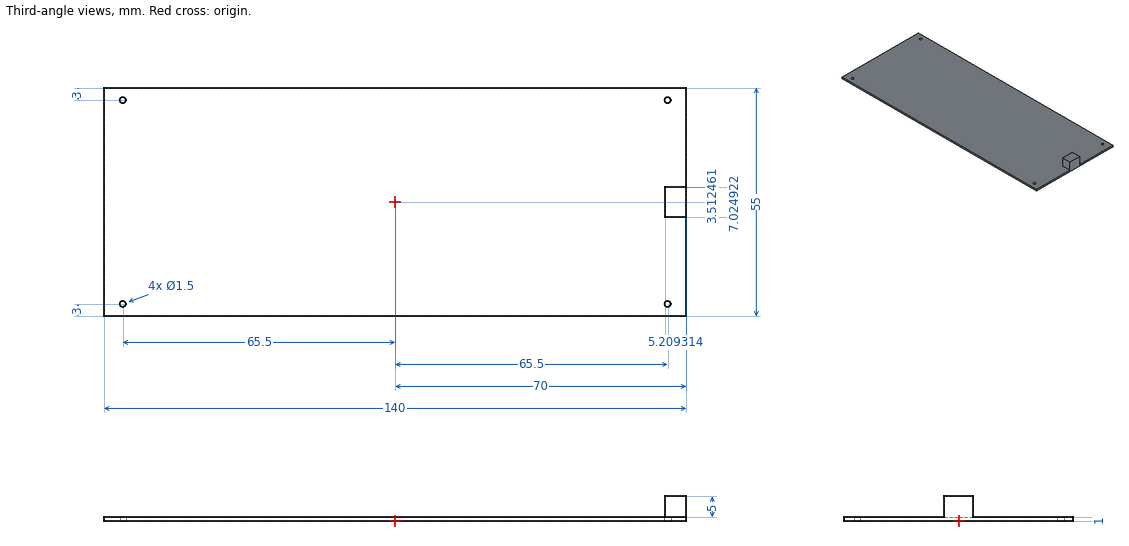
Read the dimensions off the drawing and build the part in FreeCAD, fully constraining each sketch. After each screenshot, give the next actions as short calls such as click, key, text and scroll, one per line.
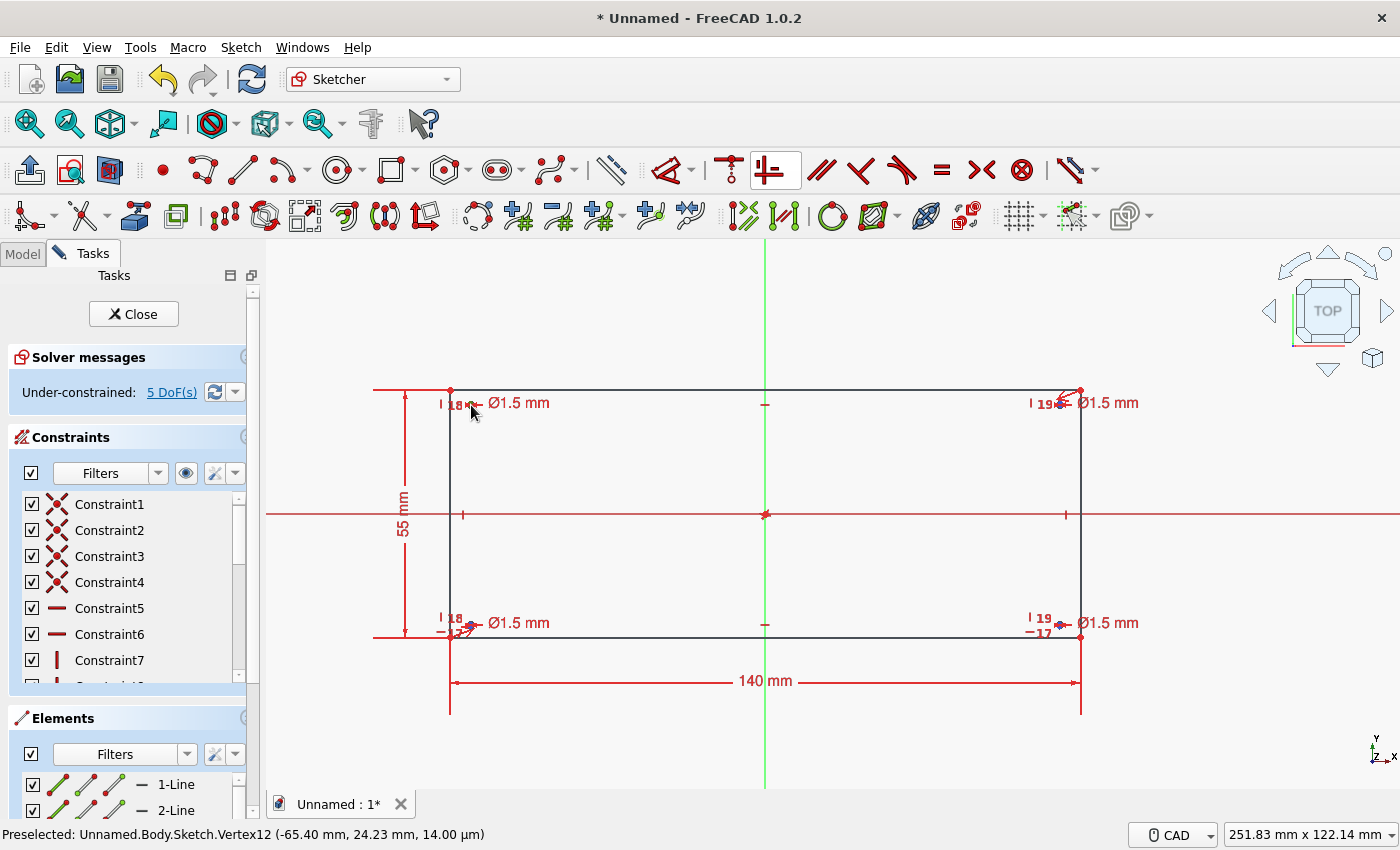
click(1060, 405)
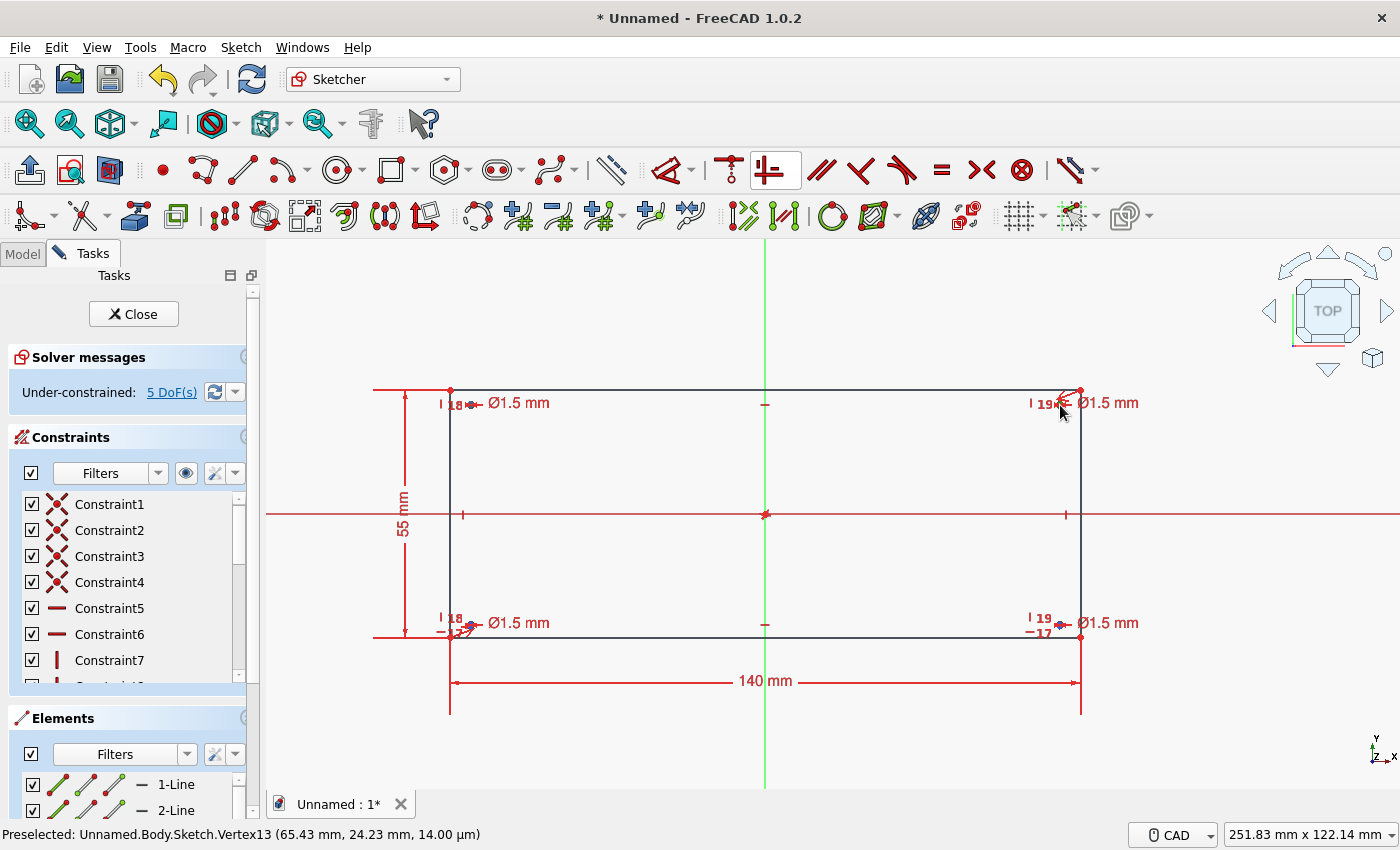
click(796, 170)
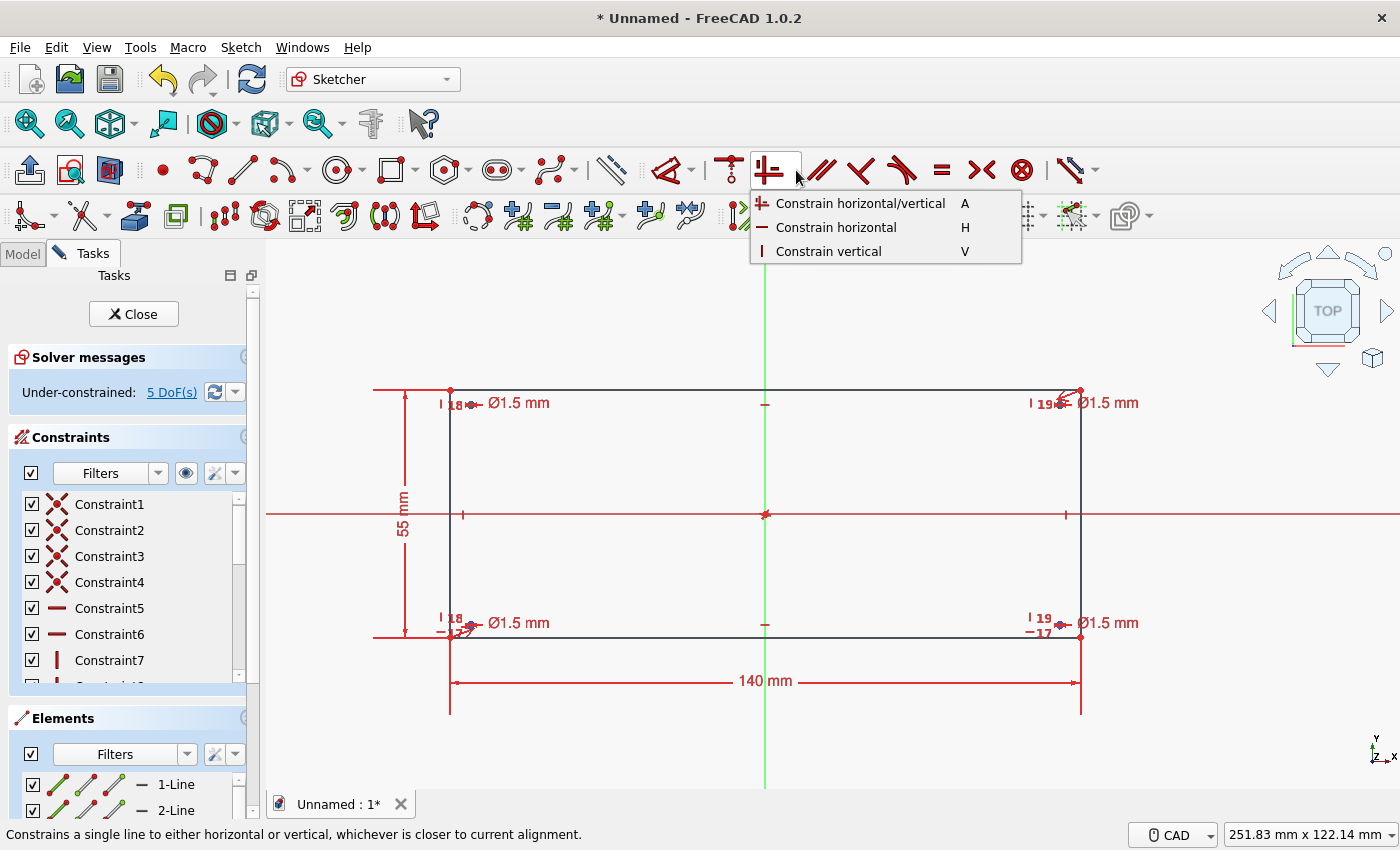
click(886, 227)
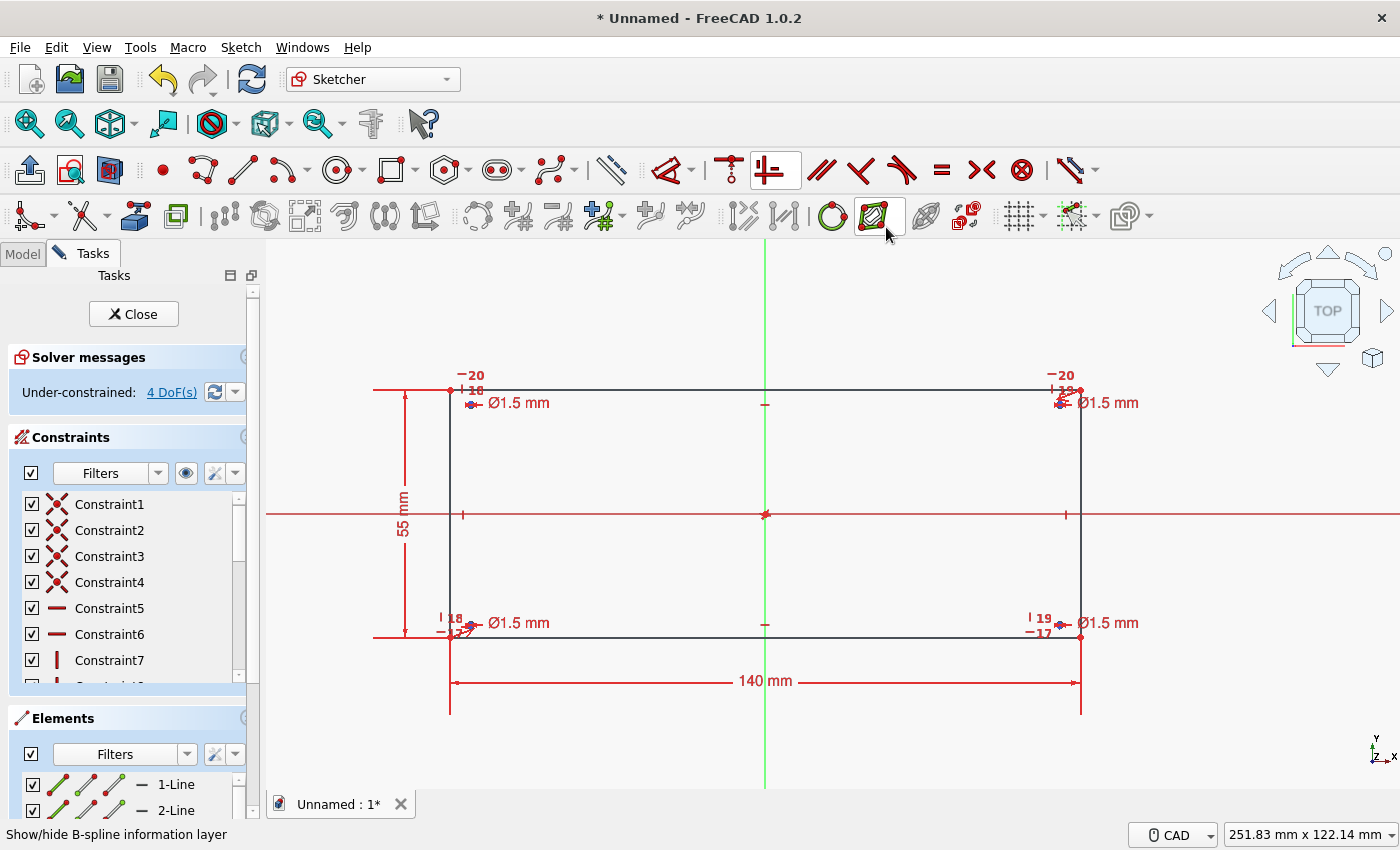
click(666, 170)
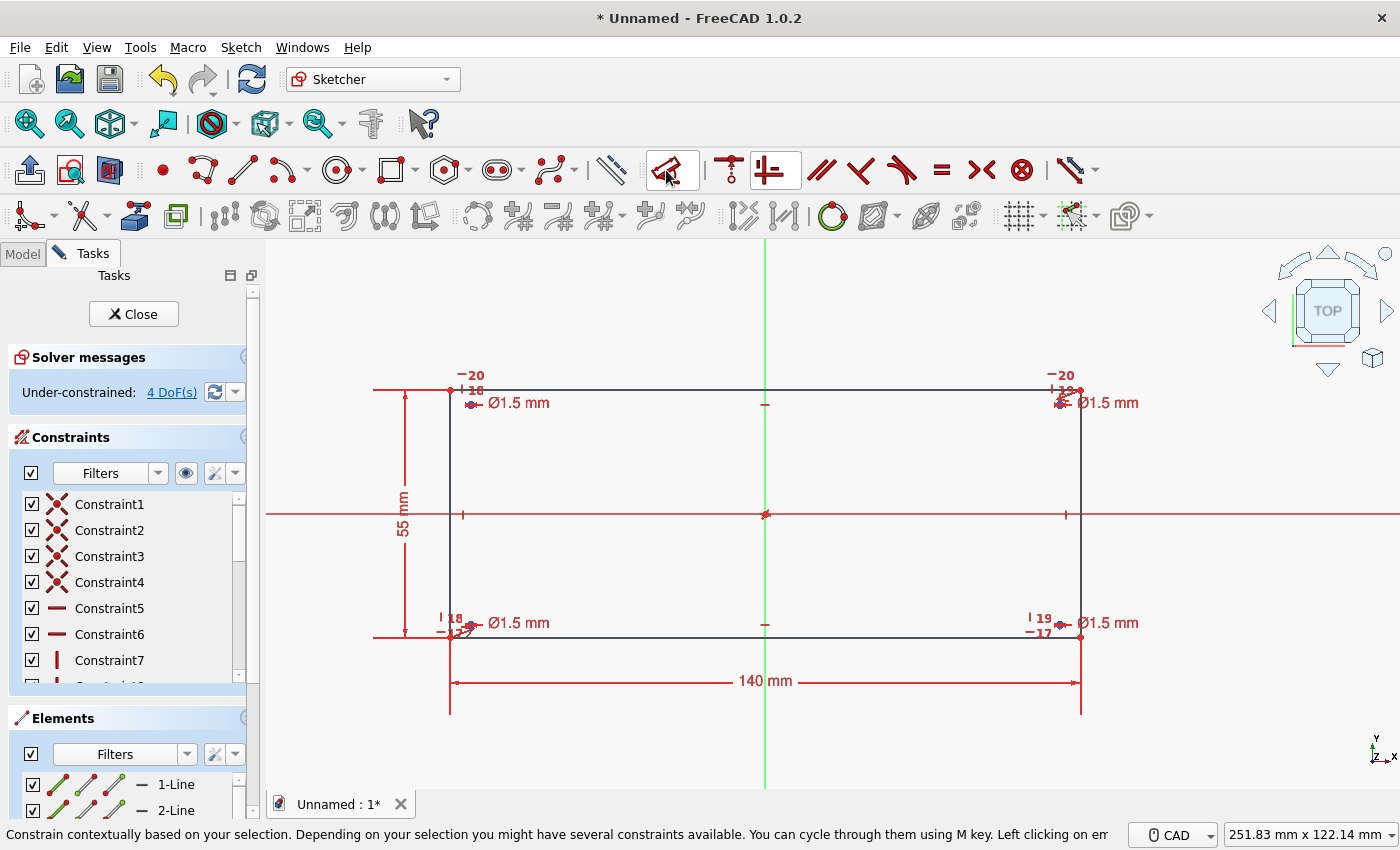
scroll(450, 638, up, 6)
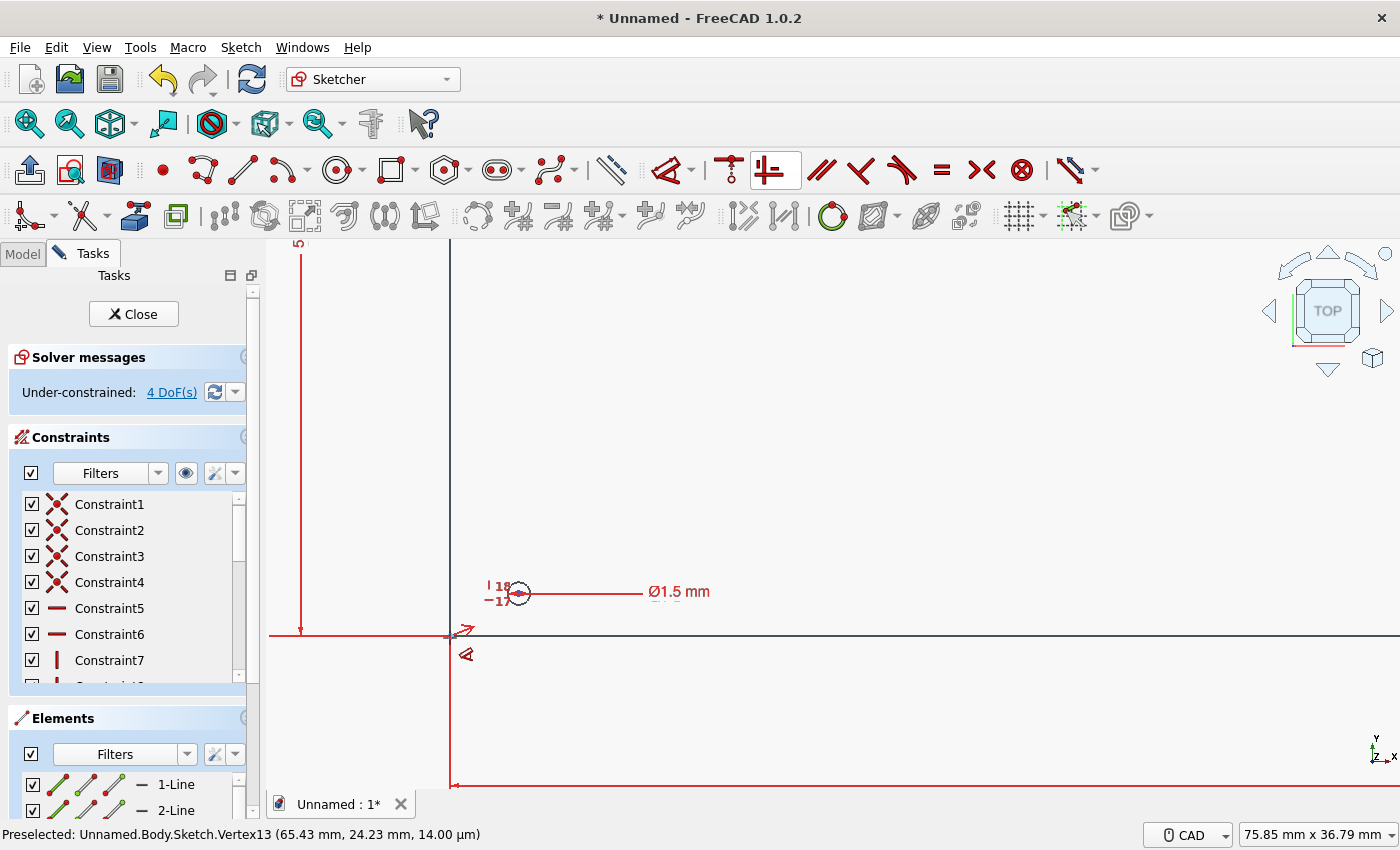
click(450, 636)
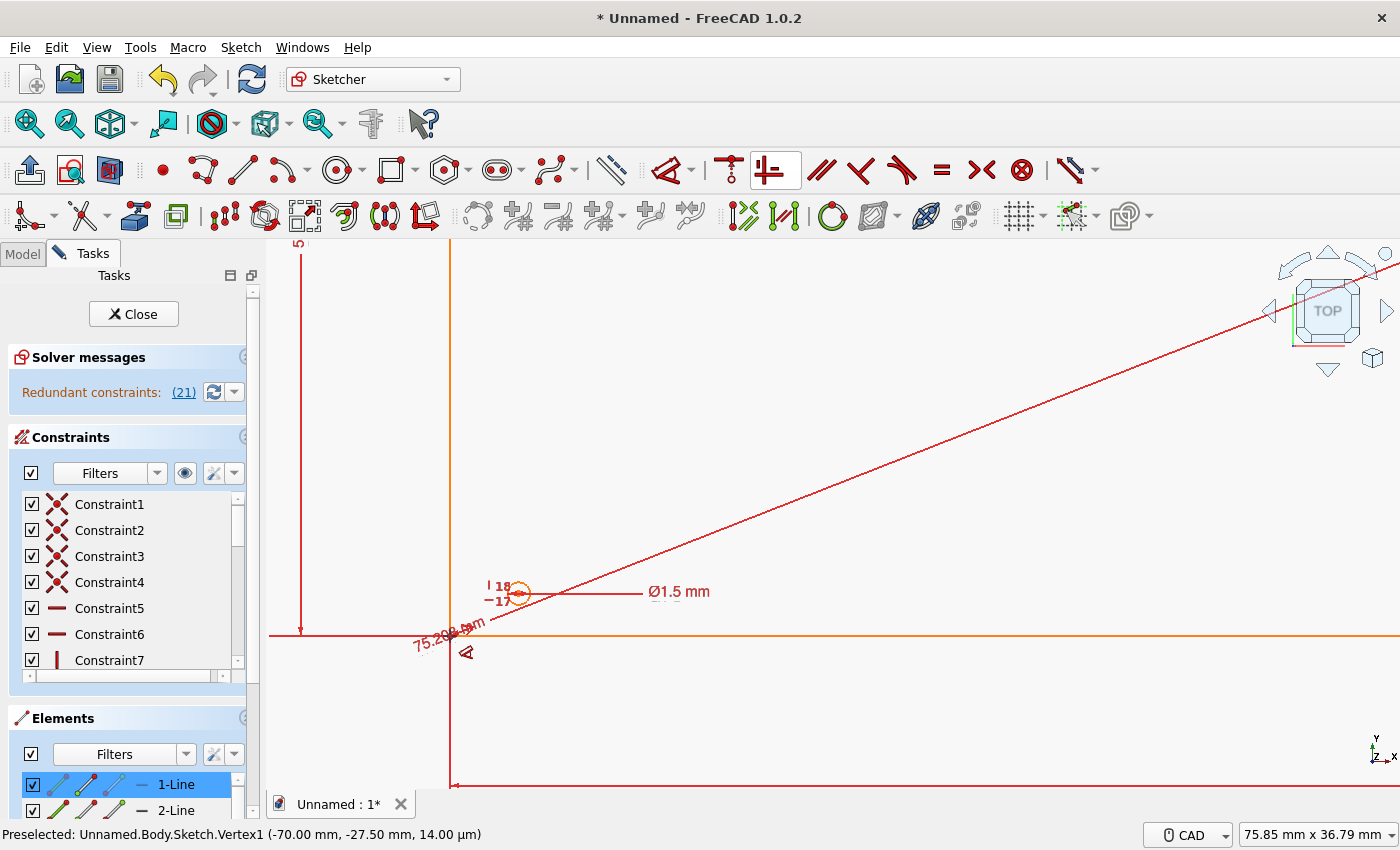
click(519, 594)
click(416, 615)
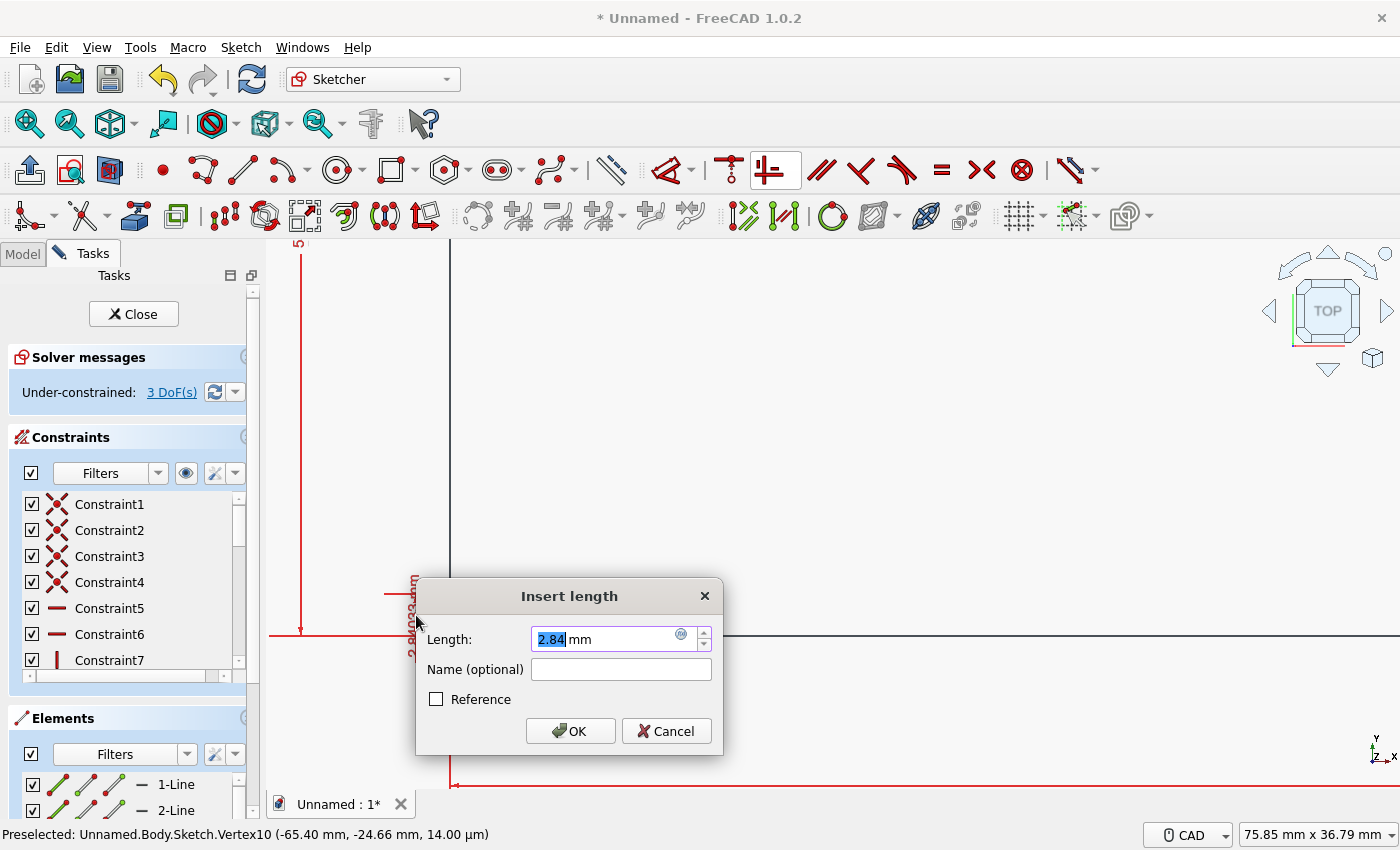
text(3)
key(Return)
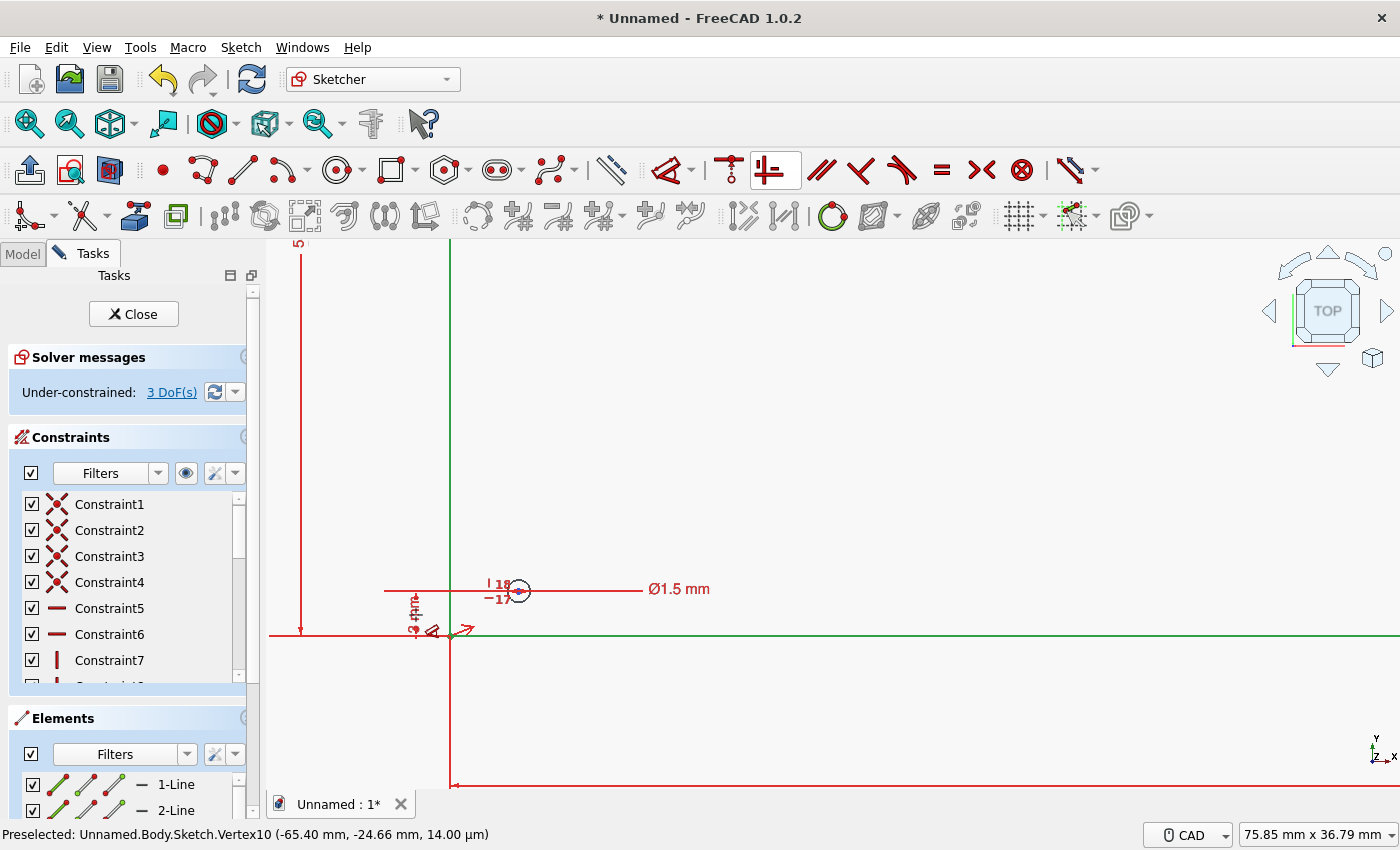
scroll(449, 639, down, 6)